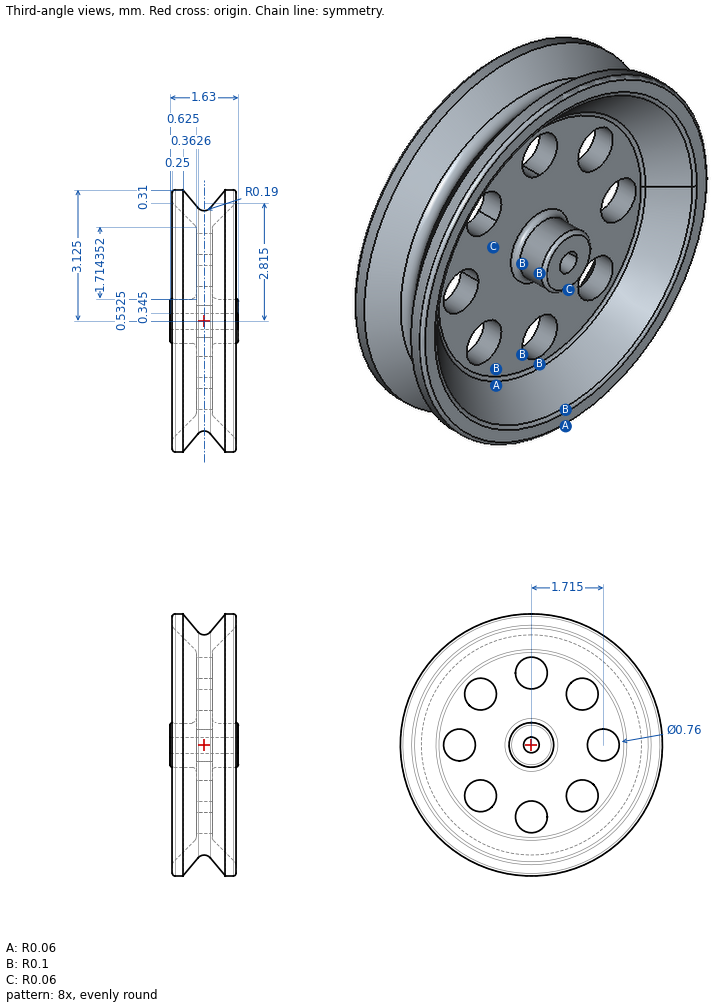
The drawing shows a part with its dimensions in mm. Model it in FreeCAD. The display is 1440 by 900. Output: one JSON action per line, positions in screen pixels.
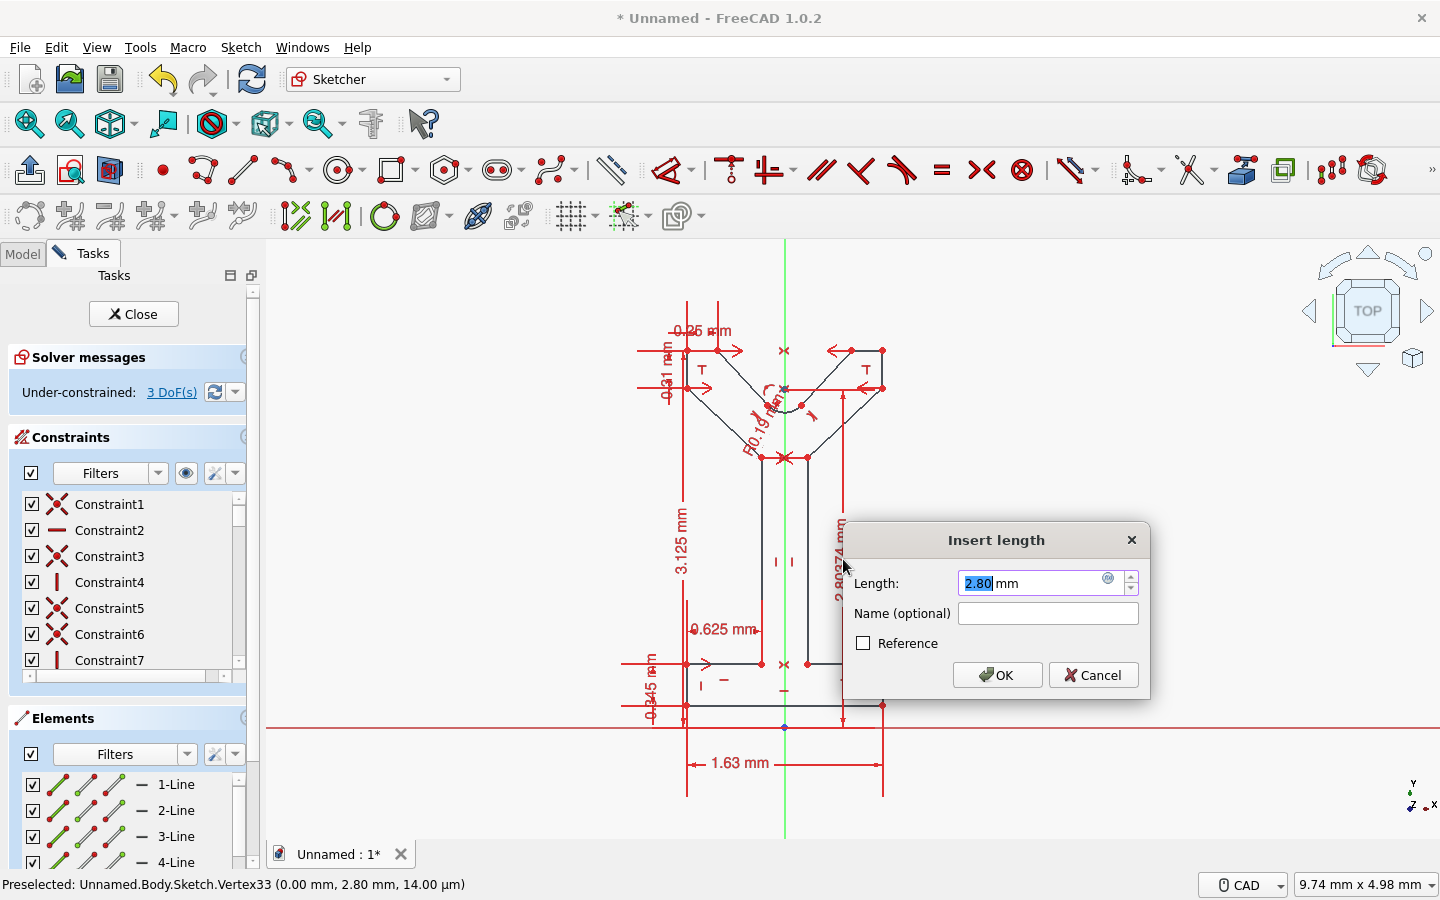
{"action": "type", "text": "2.815"}
{"action": "key", "text": "Return"}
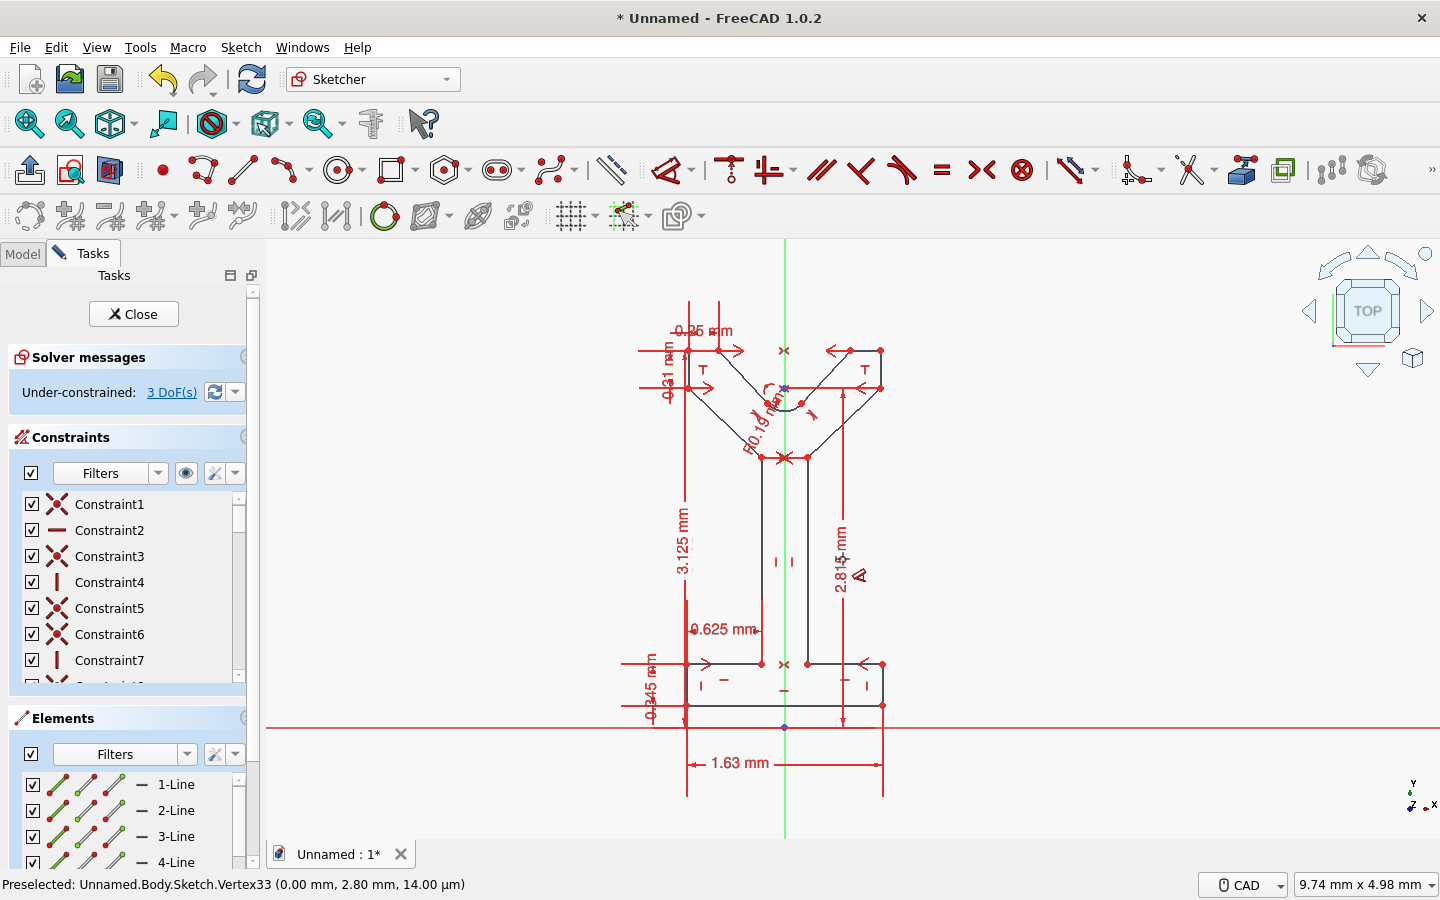
{"action": "left_click", "coordinate": [762, 664]}
{"action": "left_click", "coordinate": [728, 681]}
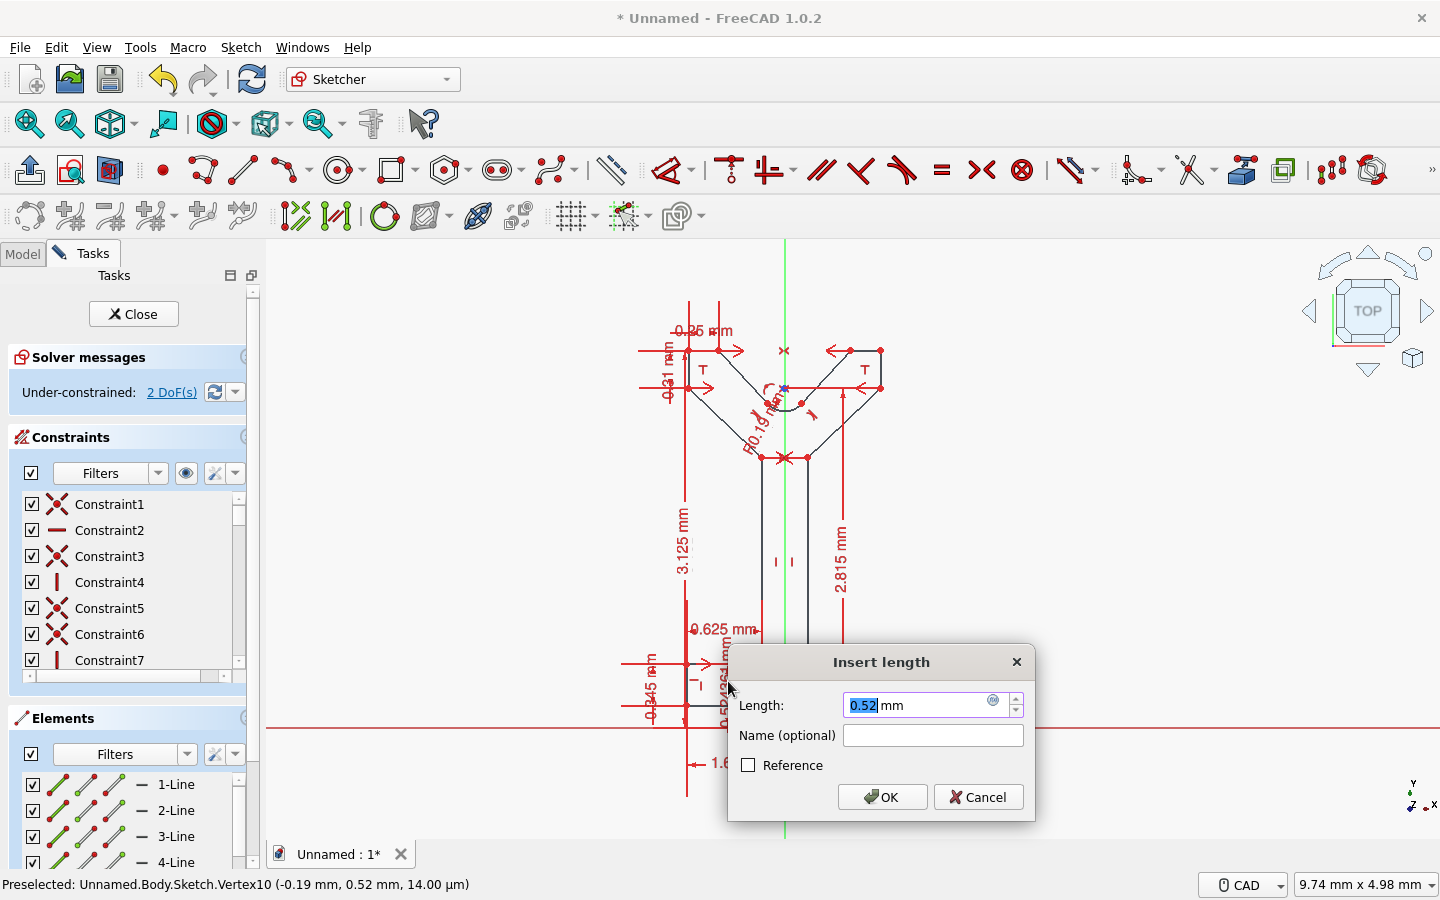
{"action": "type", "text": "0.5325"}
{"action": "key", "text": "Return"}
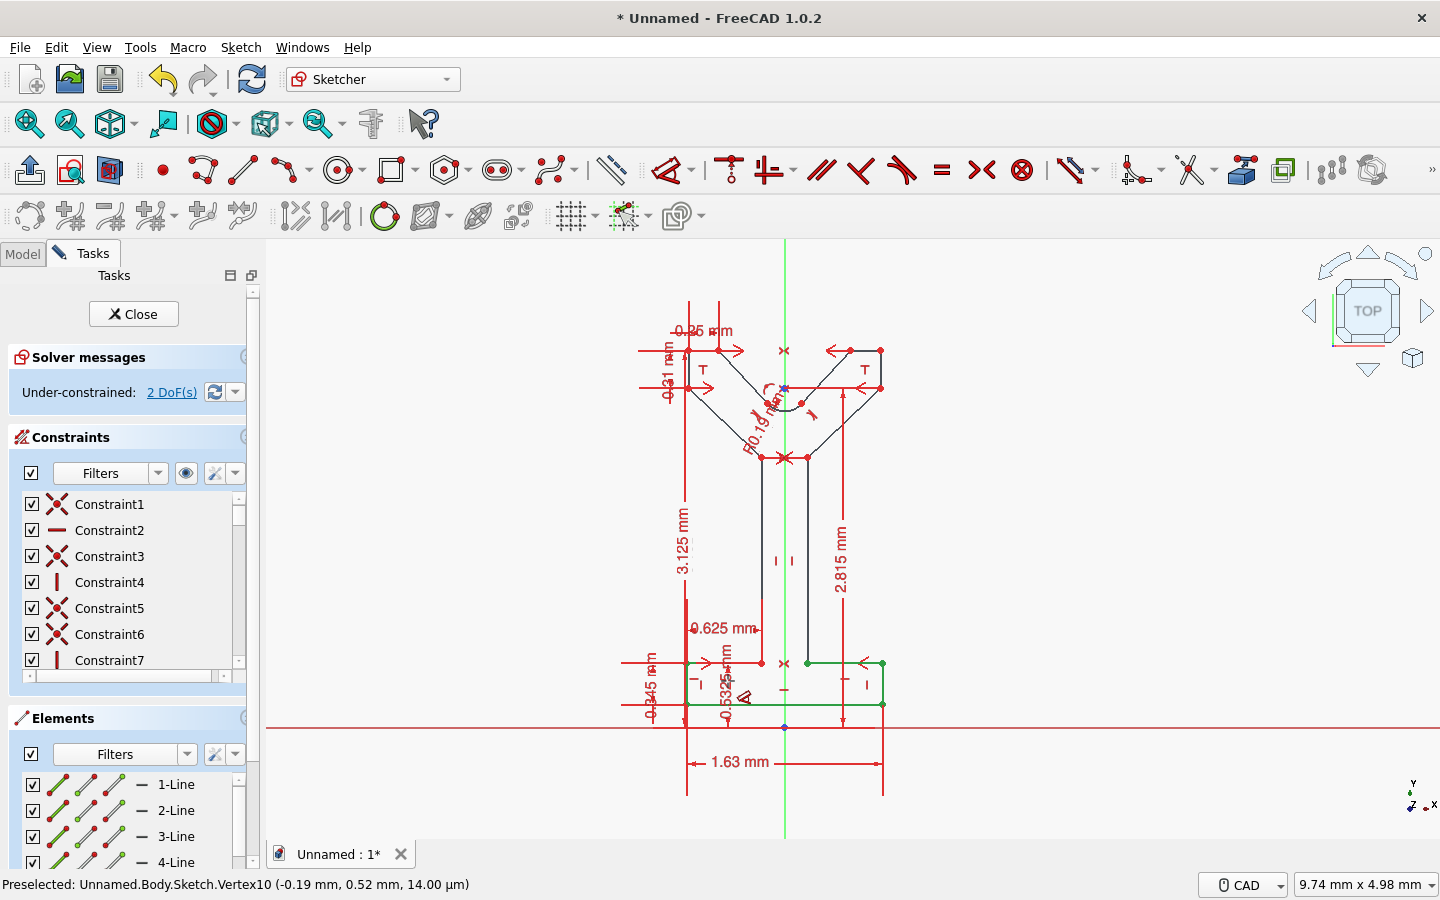
{"action": "left_click", "coordinate": [753, 388]}
{"action": "left_click", "coordinate": [743, 293]}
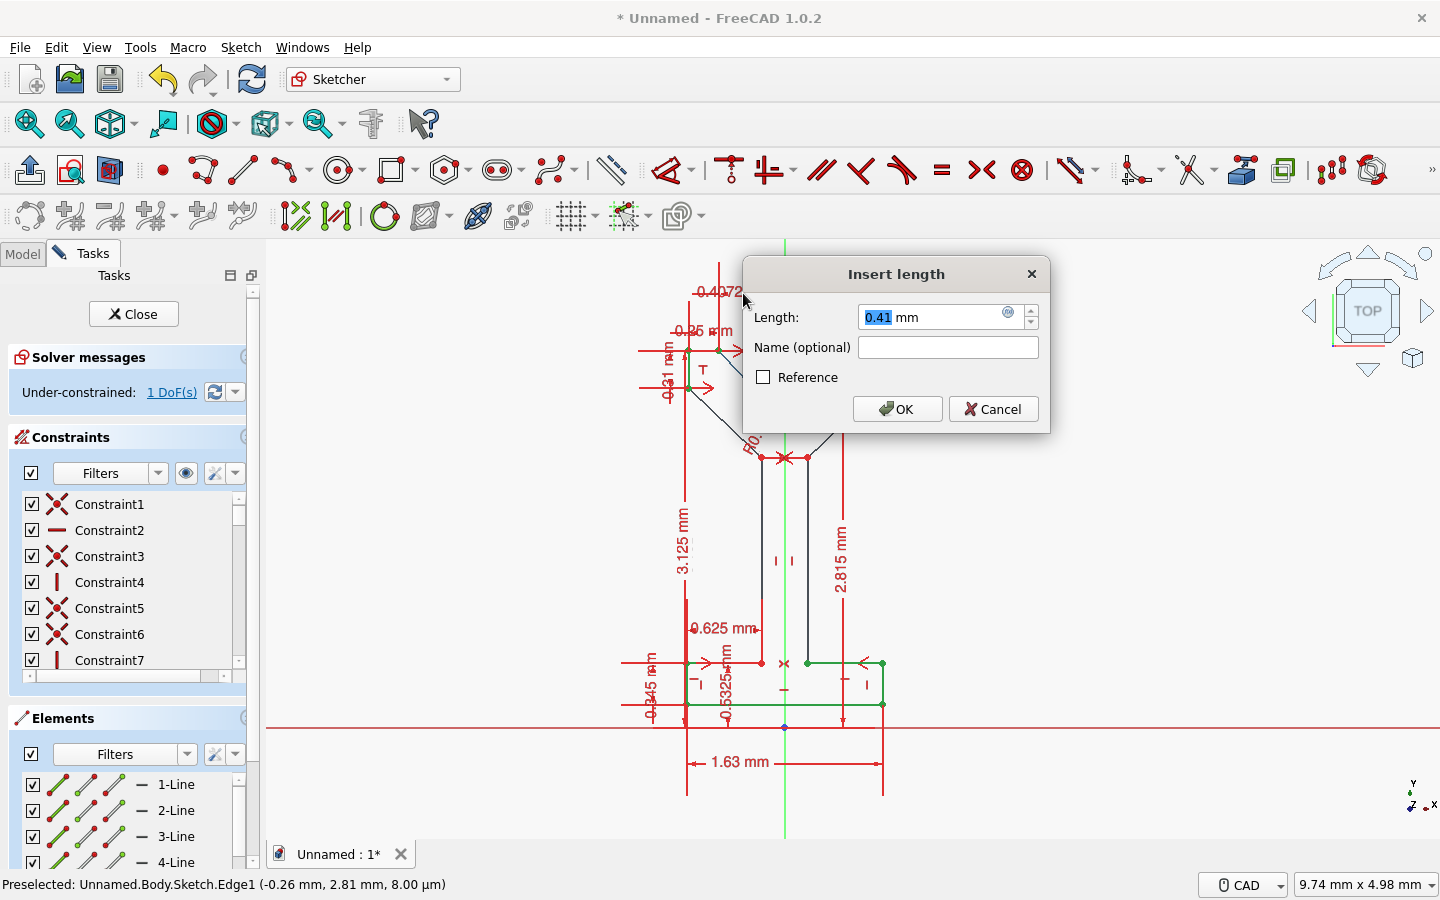
{"action": "type", "text": "0.3626"}
{"action": "key", "text": "Return"}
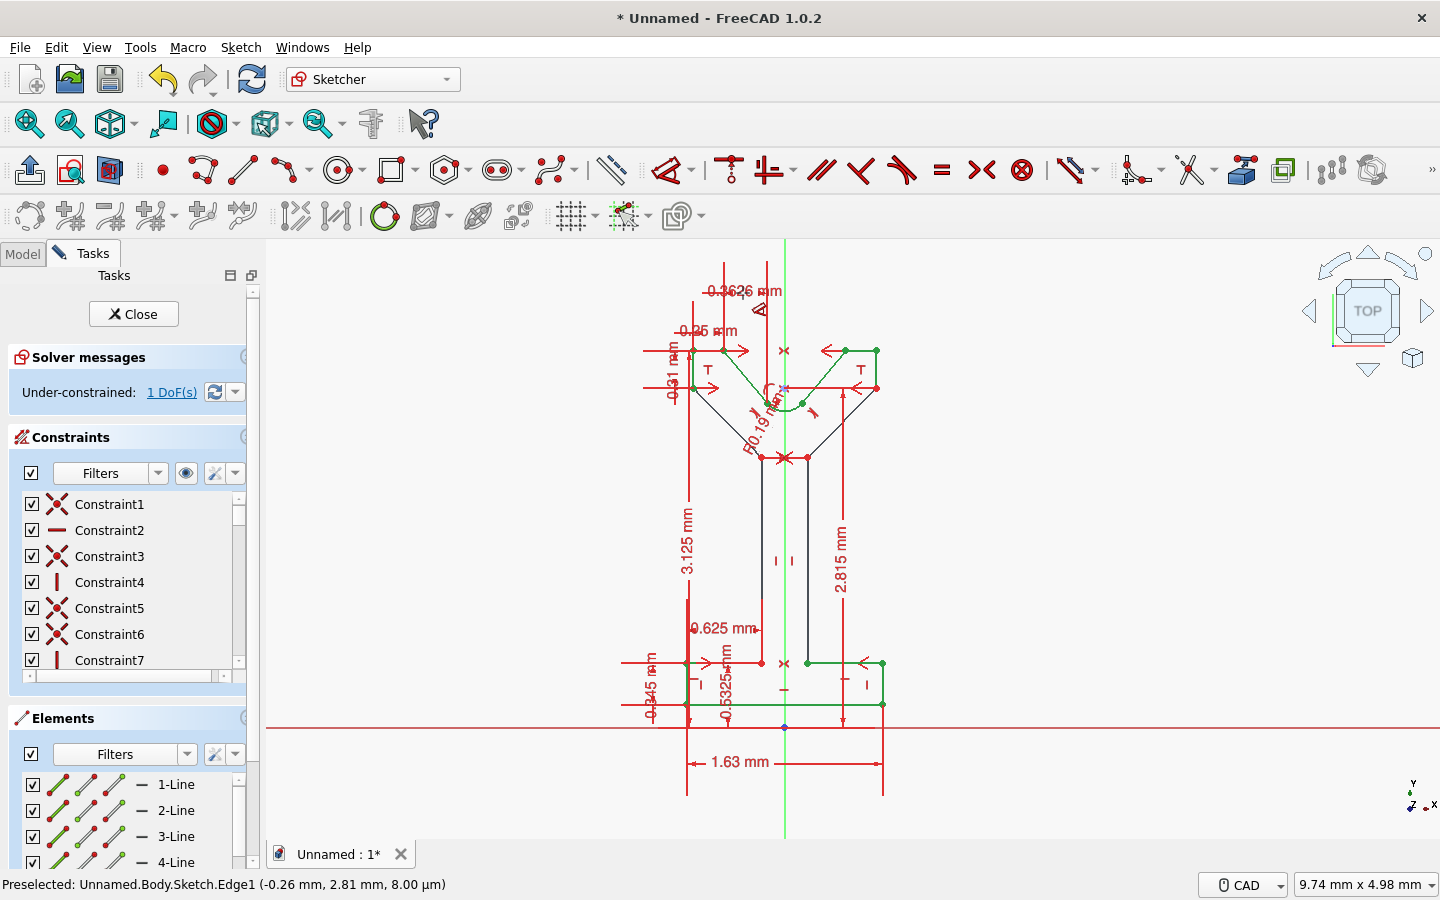
{"action": "left_click", "coordinate": [762, 520]}
{"action": "left_click", "coordinate": [728, 561]}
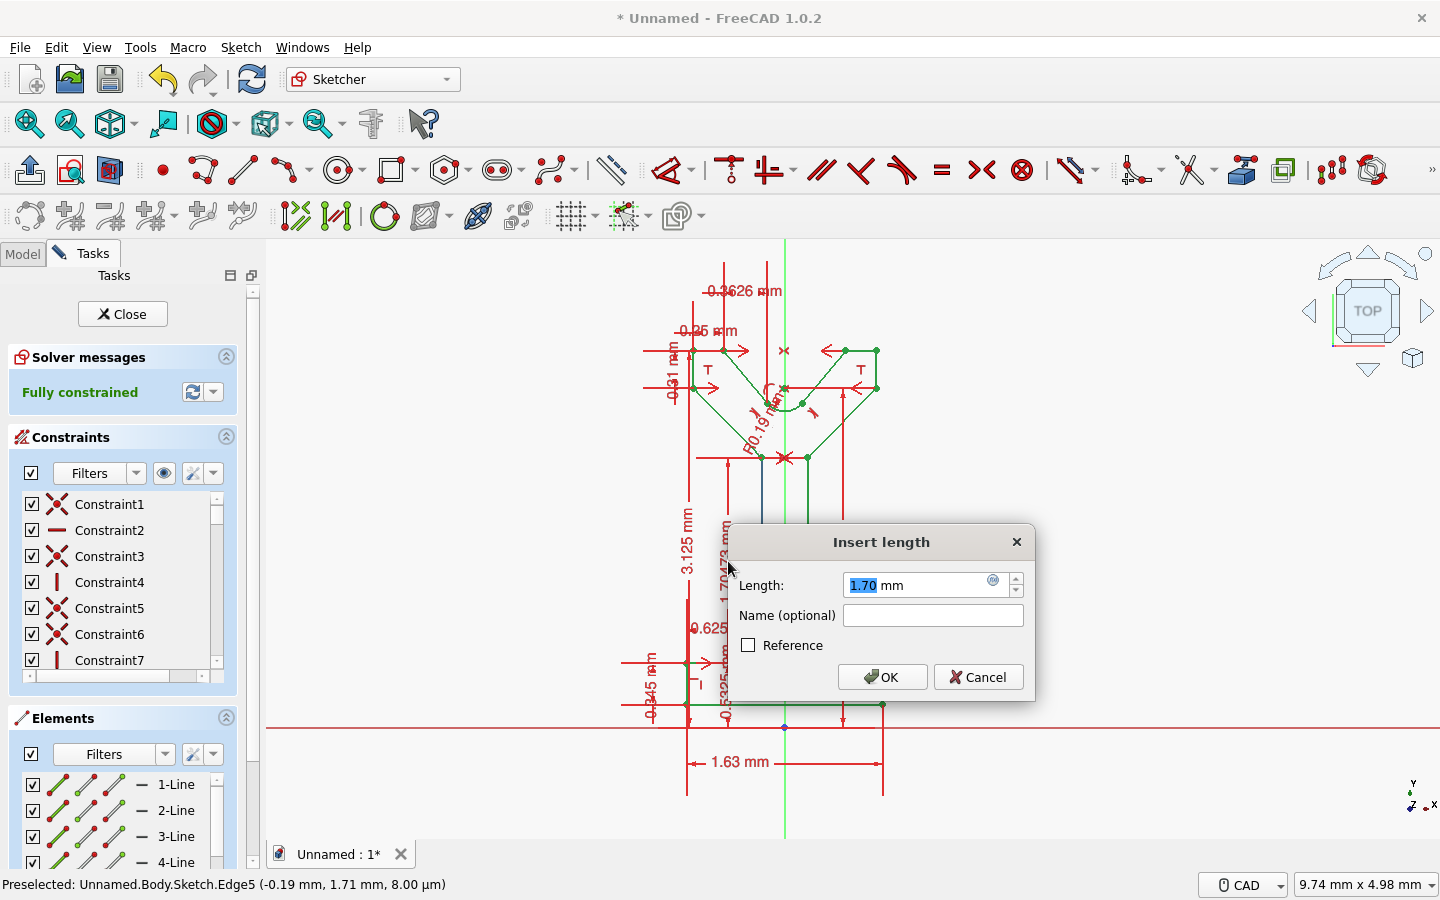
{"action": "type", "text": "1.714352"}
{"action": "key", "text": "Return"}
{"action": "key", "text": "Escape"}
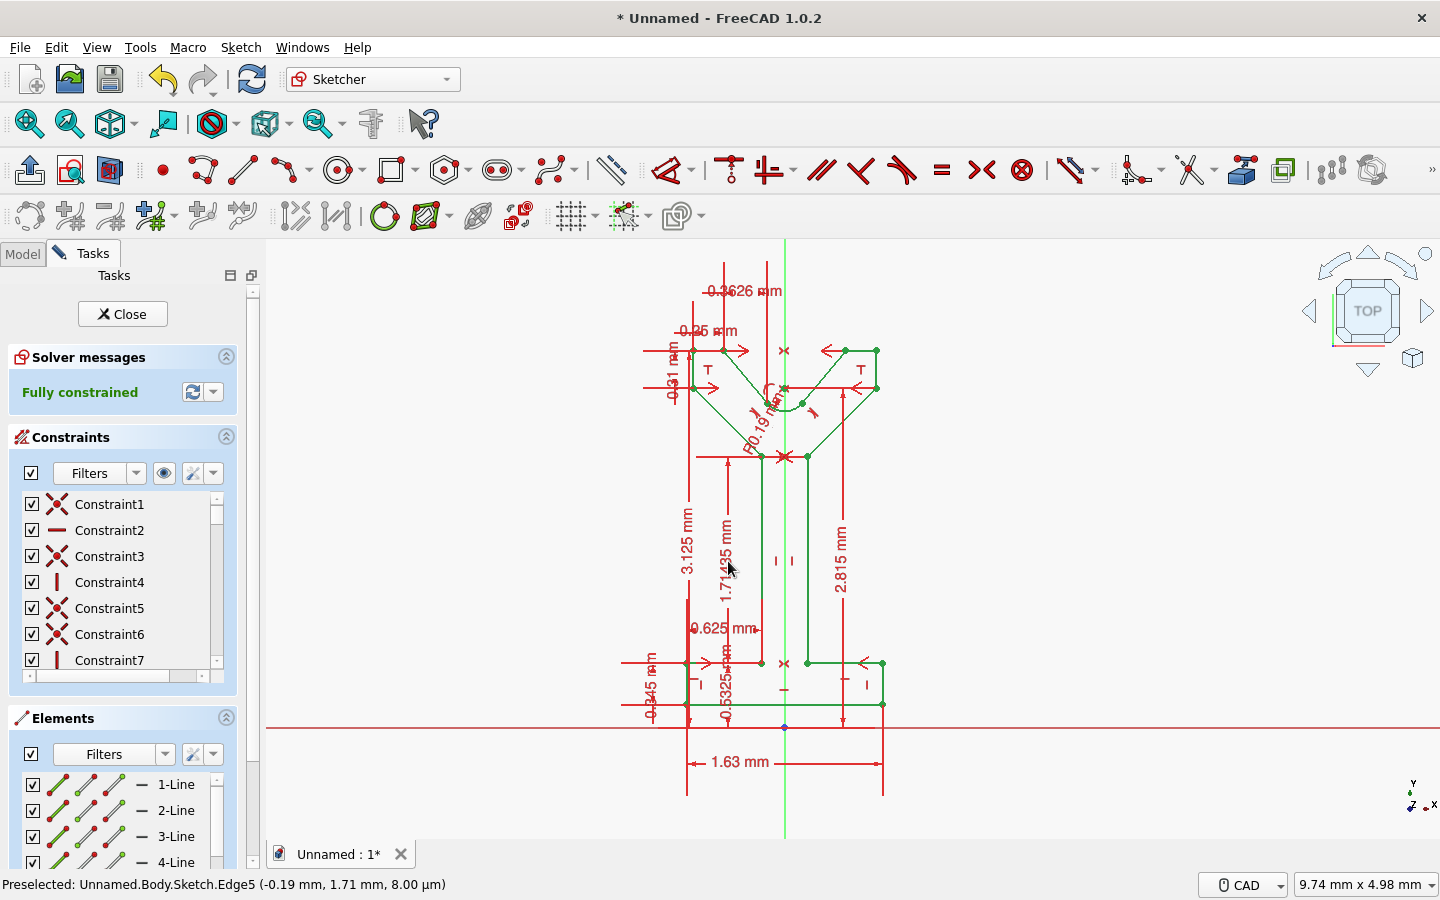
{"action": "left_click", "coordinate": [123, 314]}